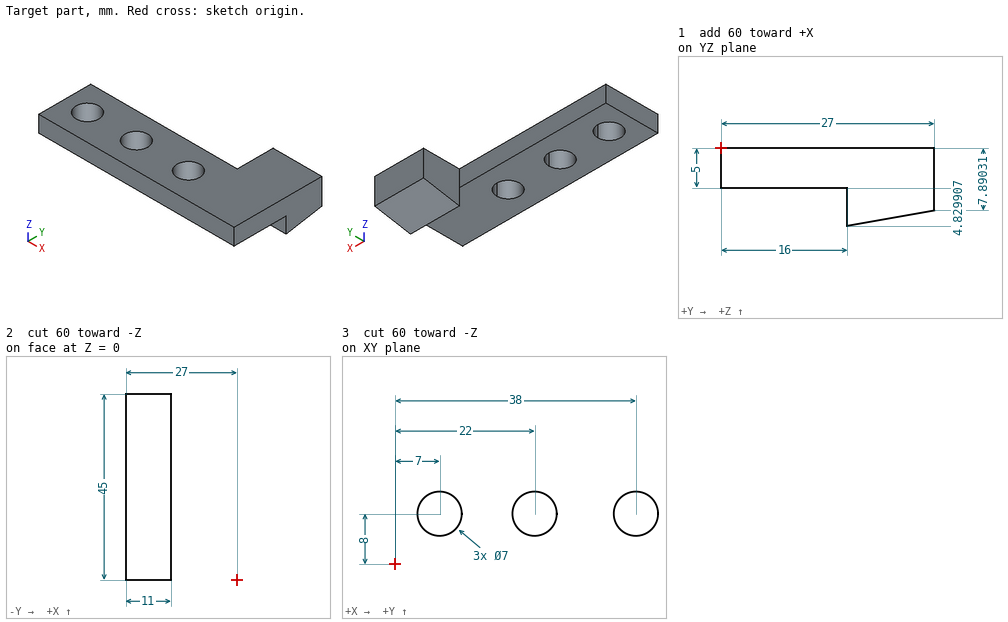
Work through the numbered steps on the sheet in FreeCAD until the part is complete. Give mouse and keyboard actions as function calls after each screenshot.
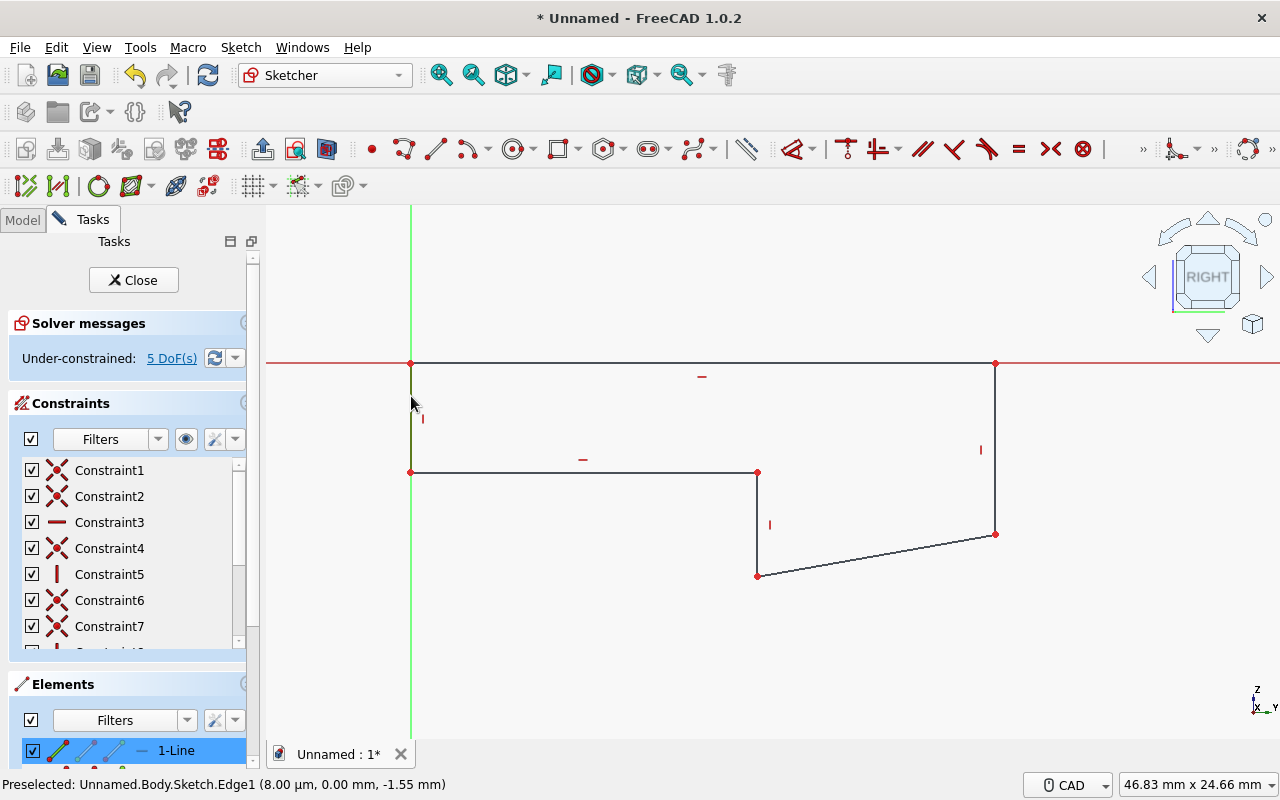
click(814, 150)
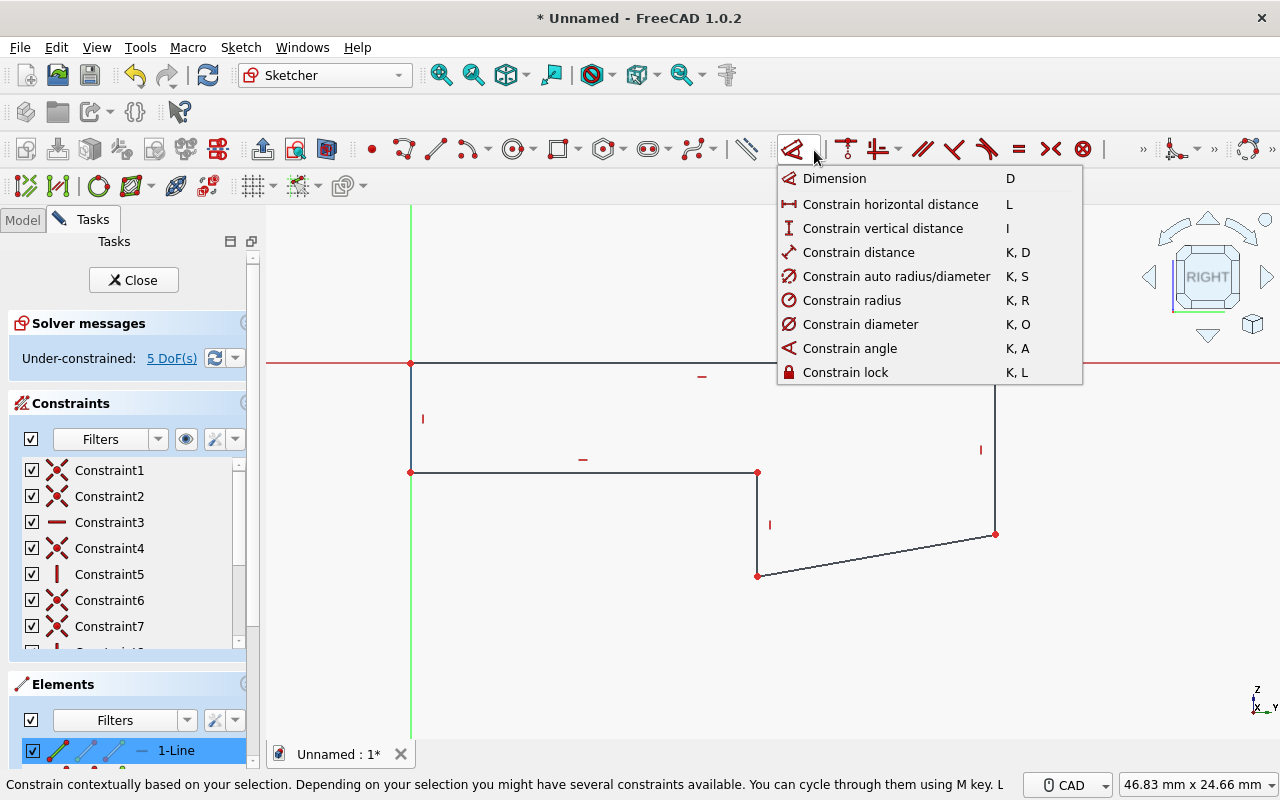
click(930, 228)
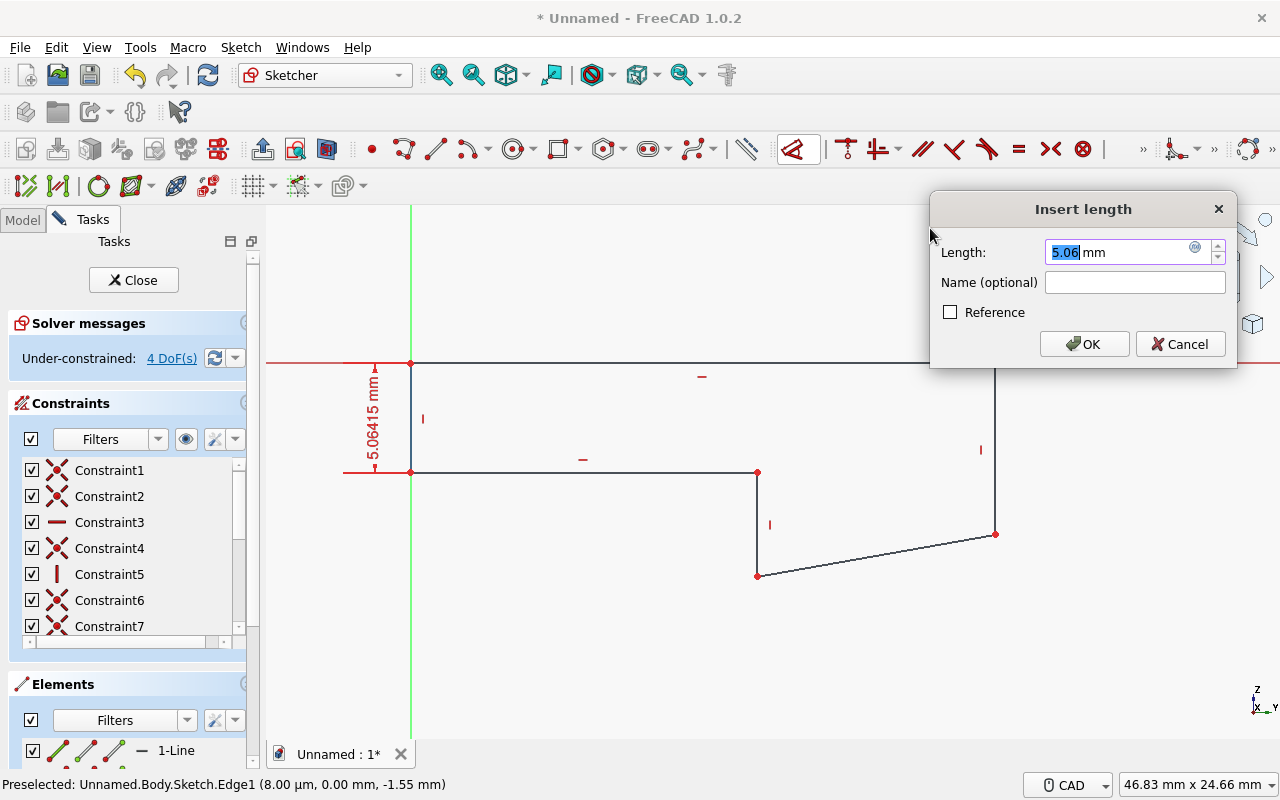
text(5)
key(Return)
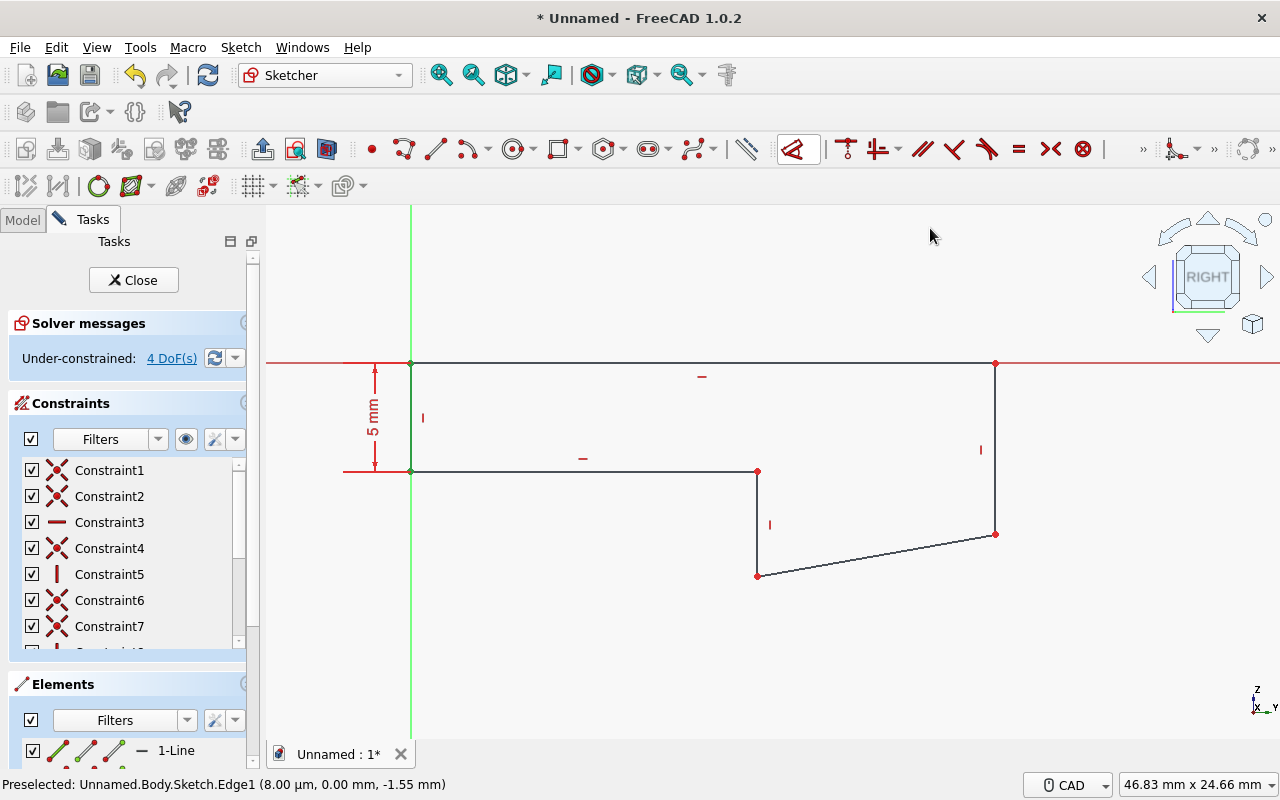
click(515, 472)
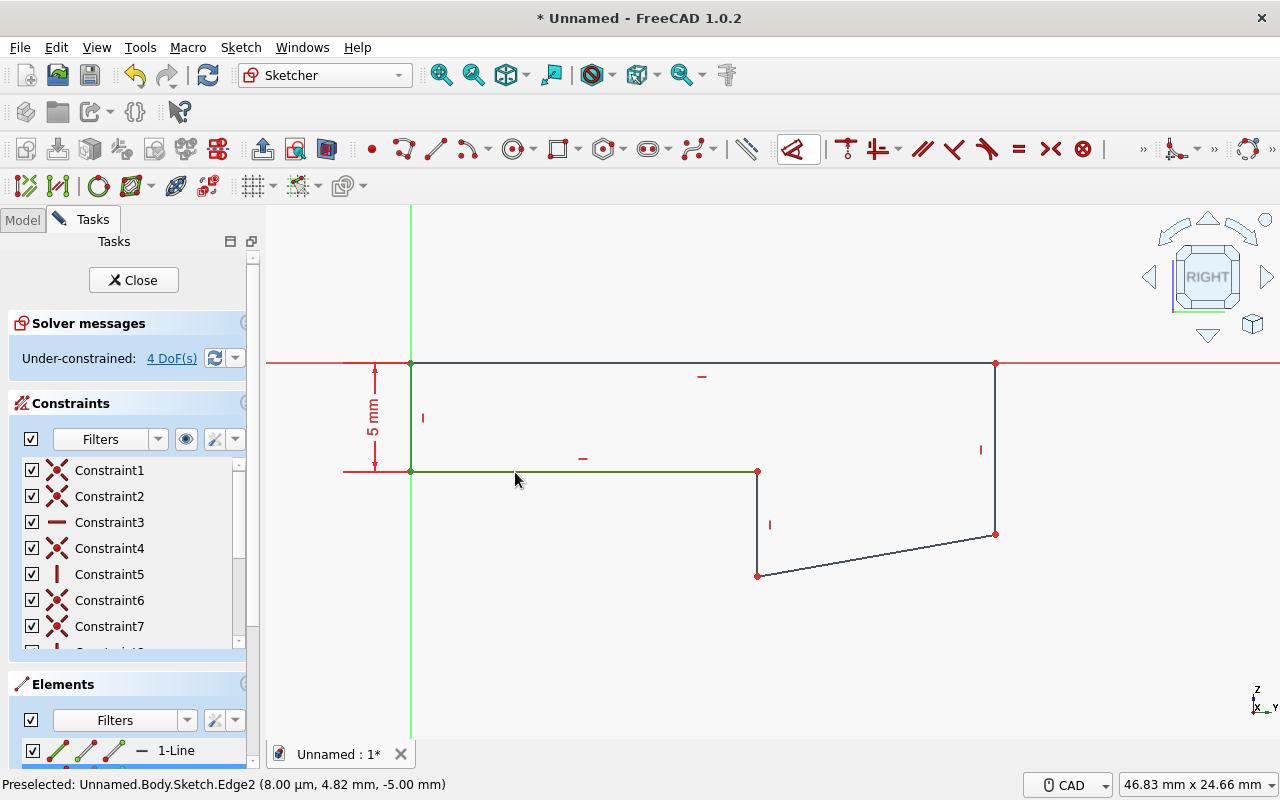
key(l)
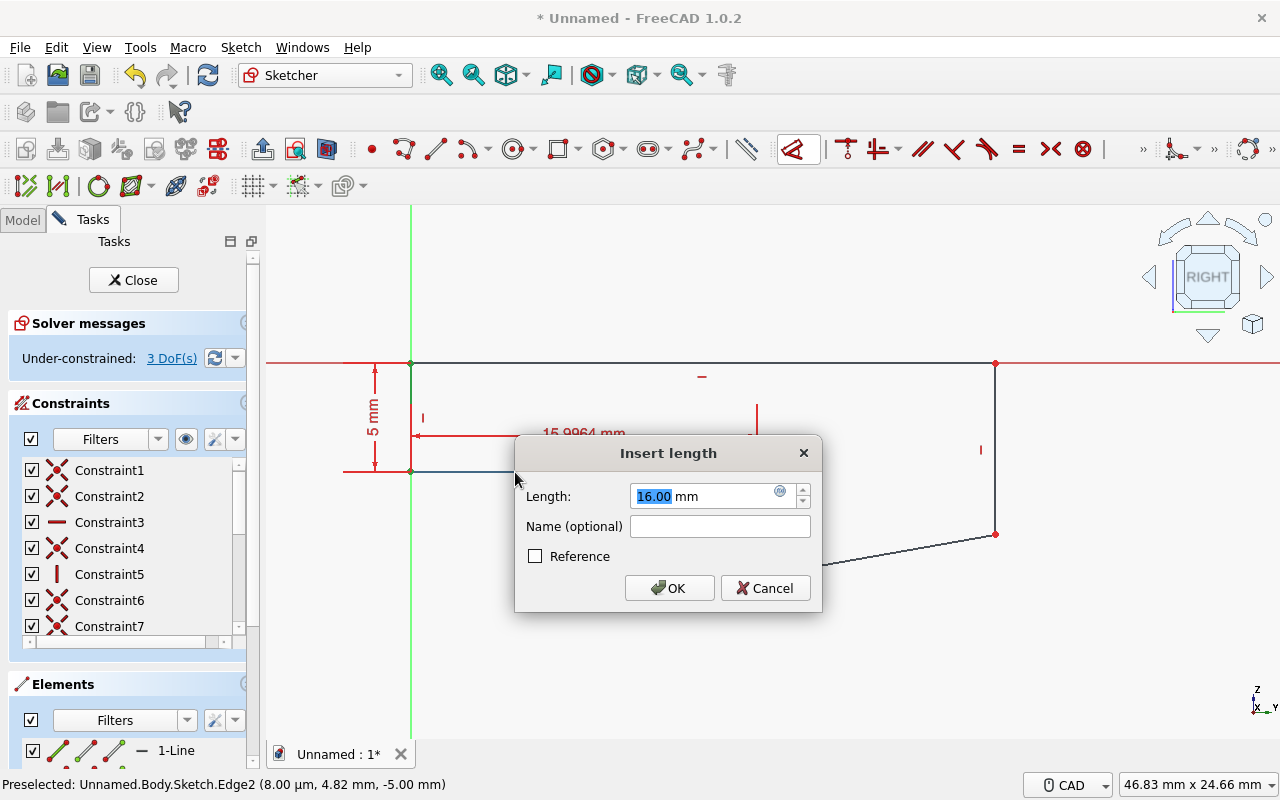
text(16)
key(Return)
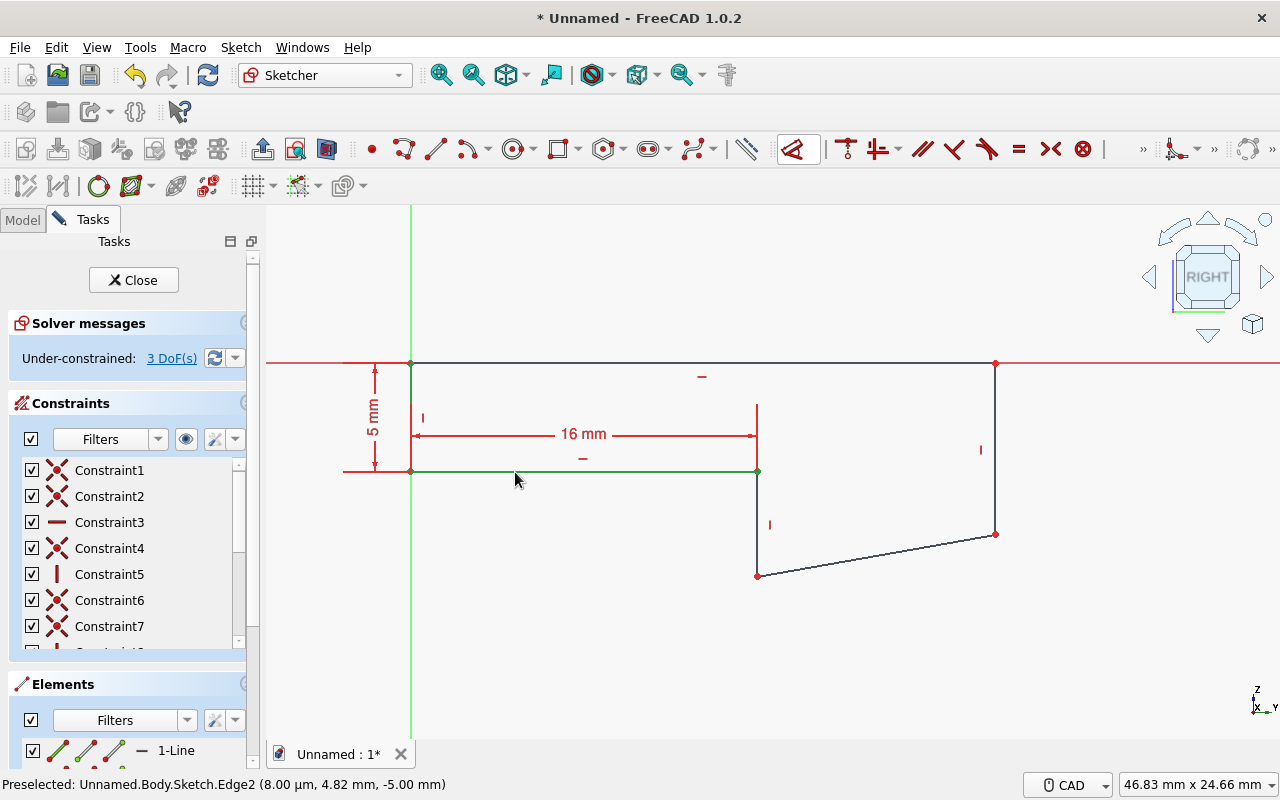
click(820, 363)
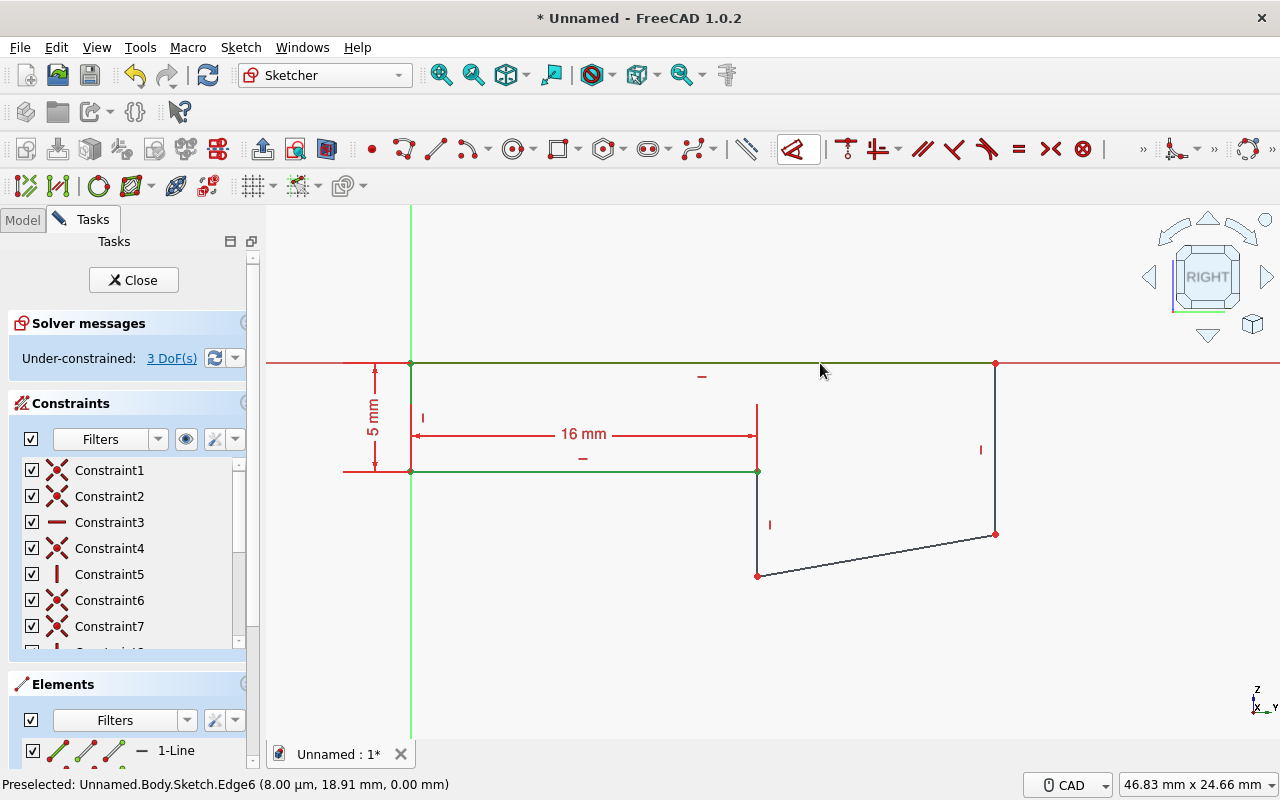
key(l)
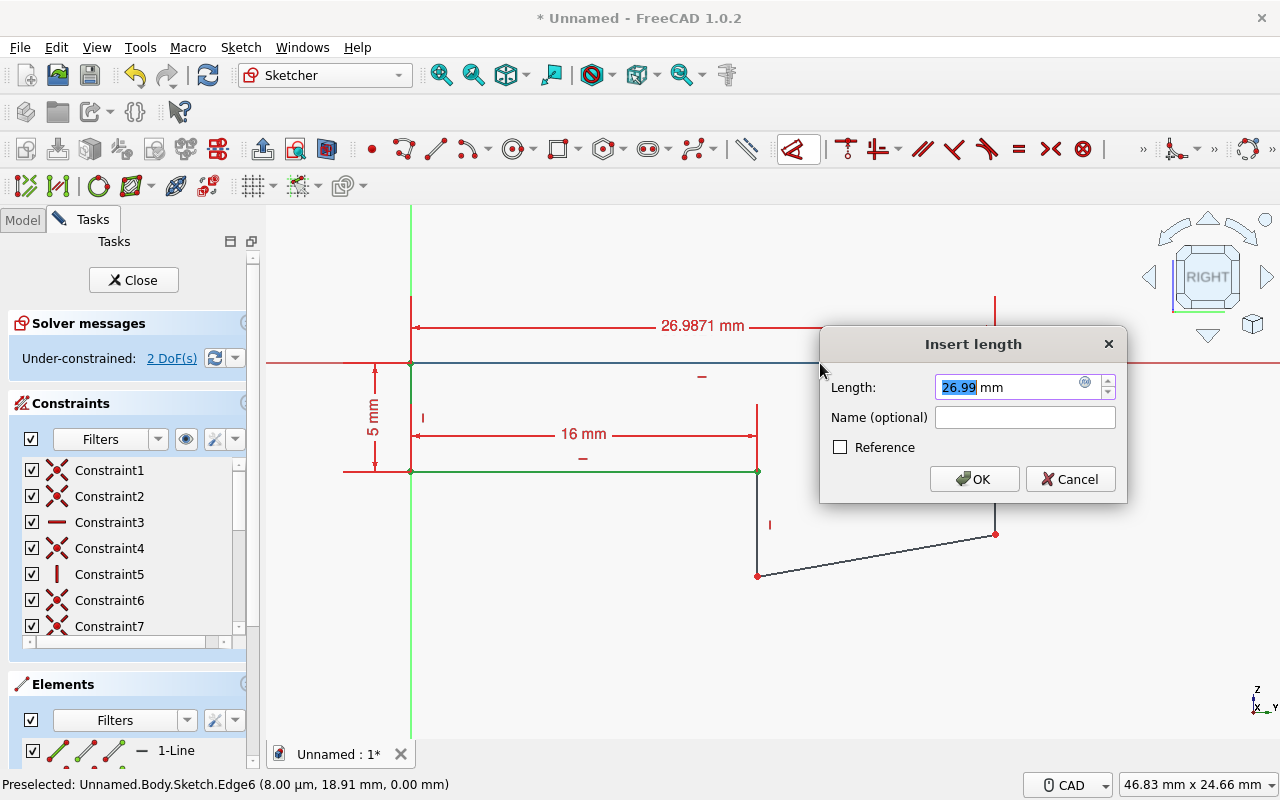
text(27)
key(Return)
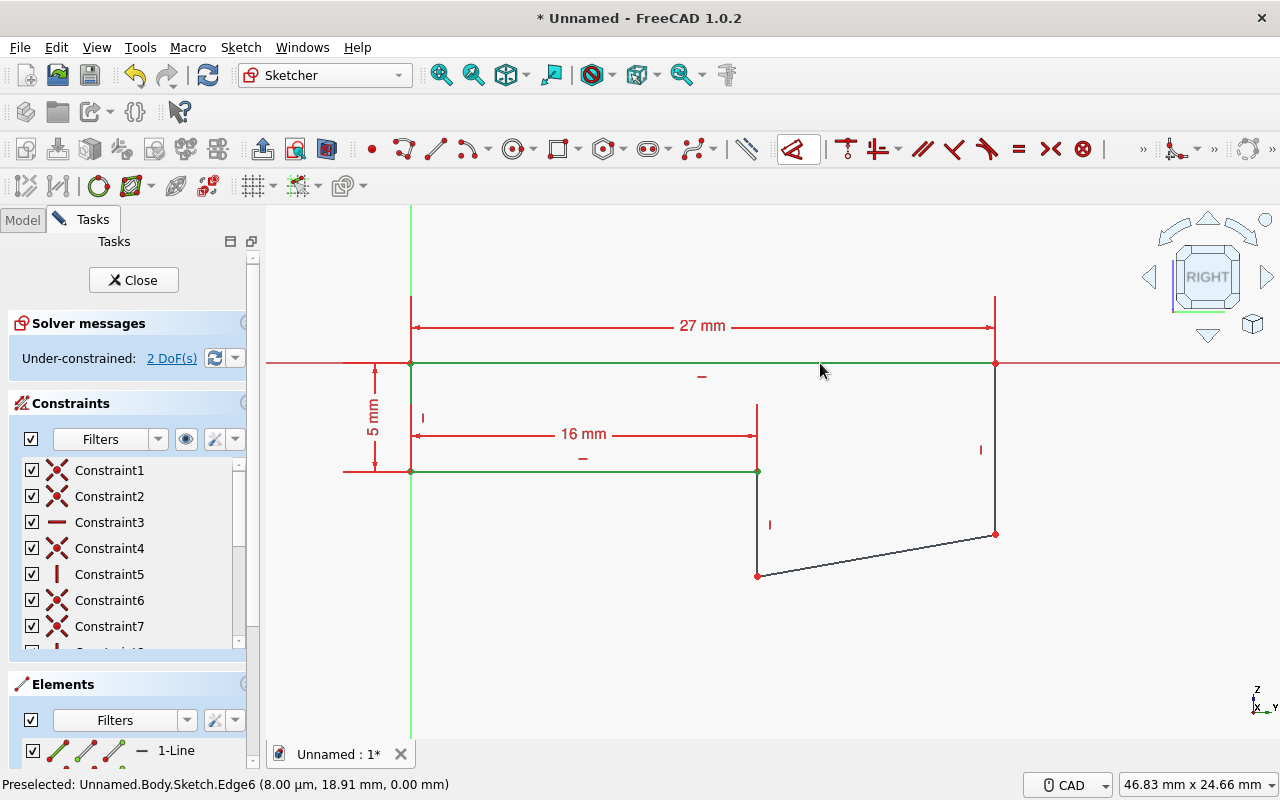
click(995, 484)